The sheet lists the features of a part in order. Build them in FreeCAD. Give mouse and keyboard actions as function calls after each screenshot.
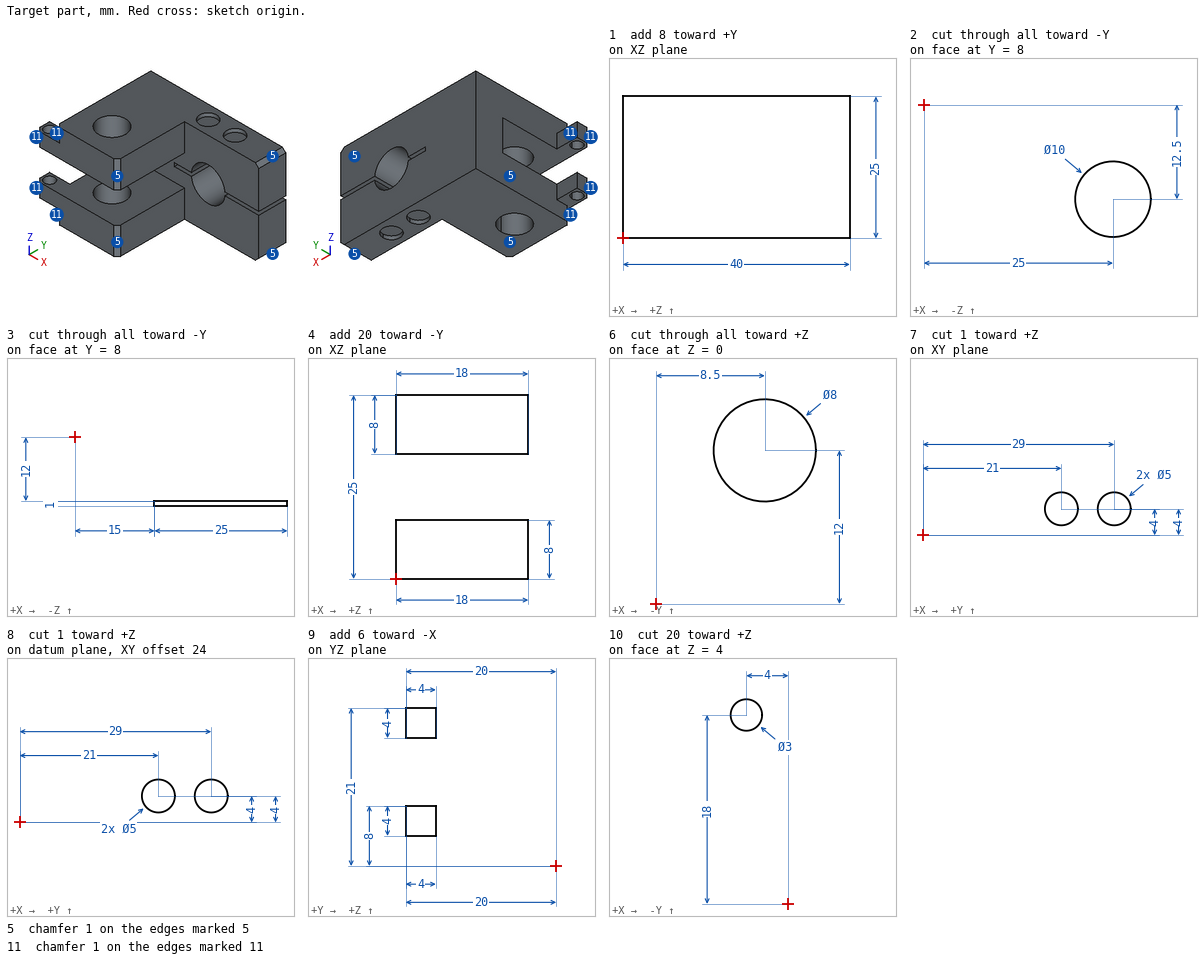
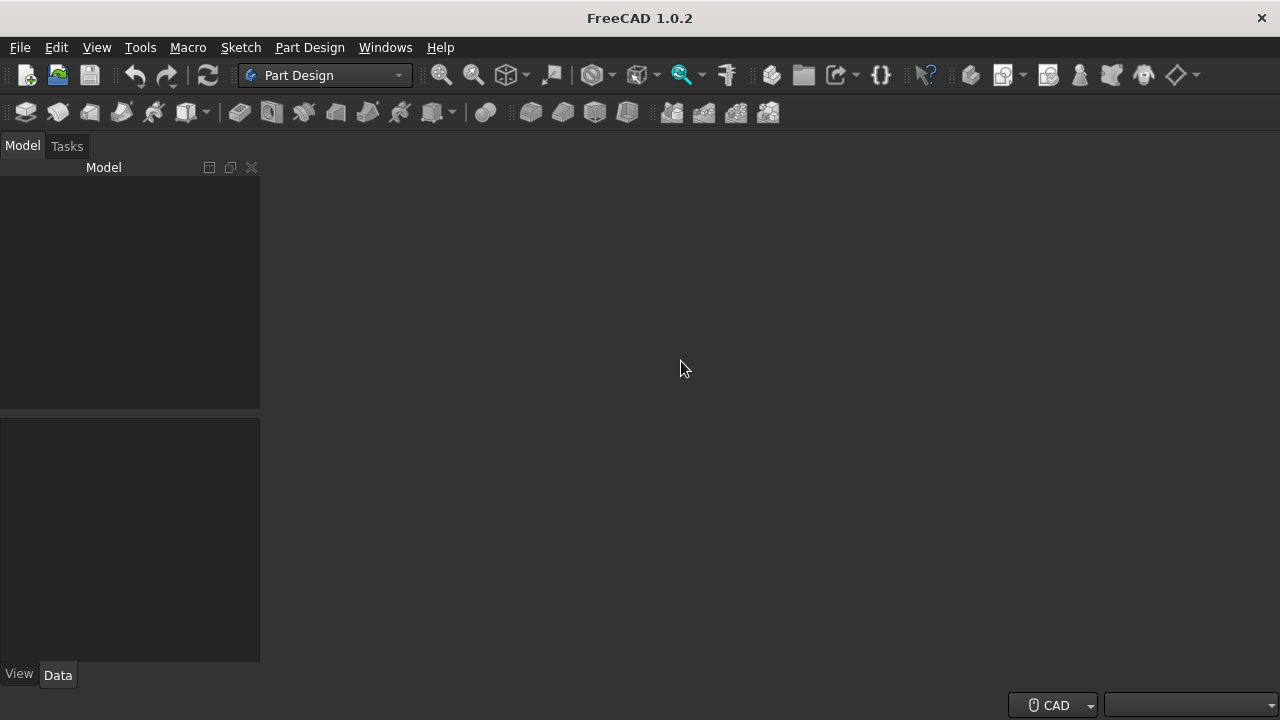
click(26, 76)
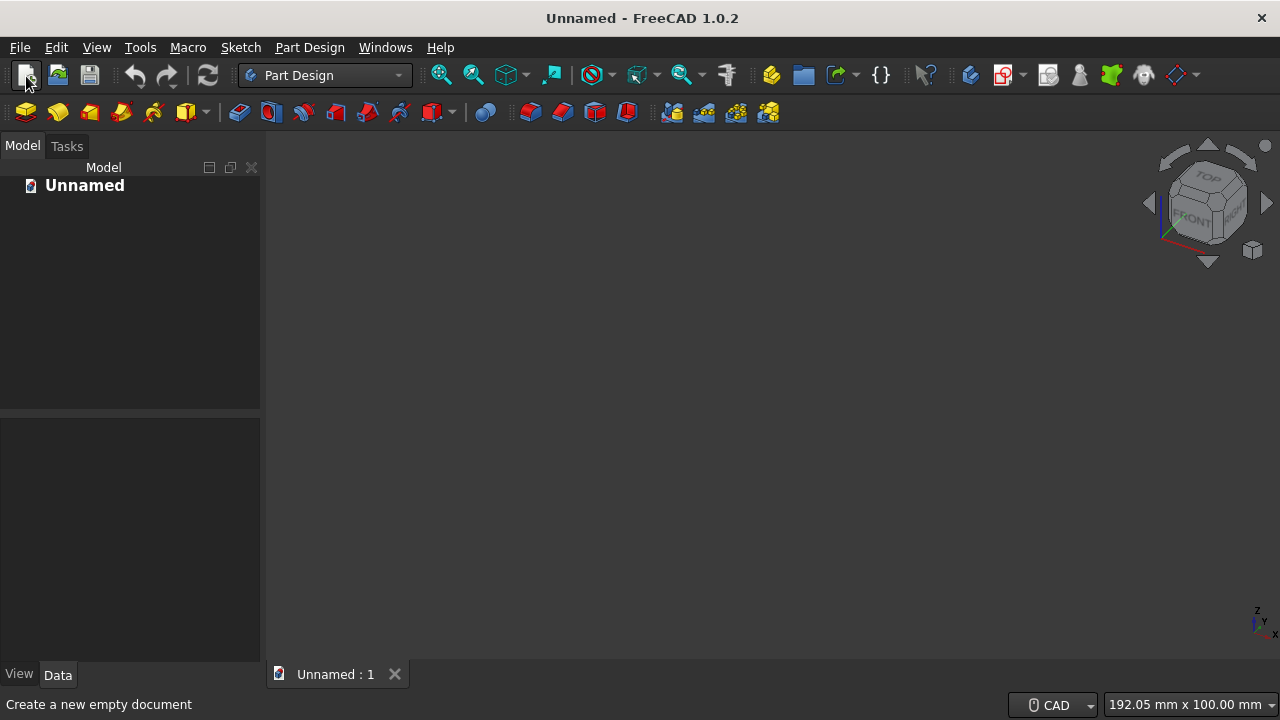
click(1004, 76)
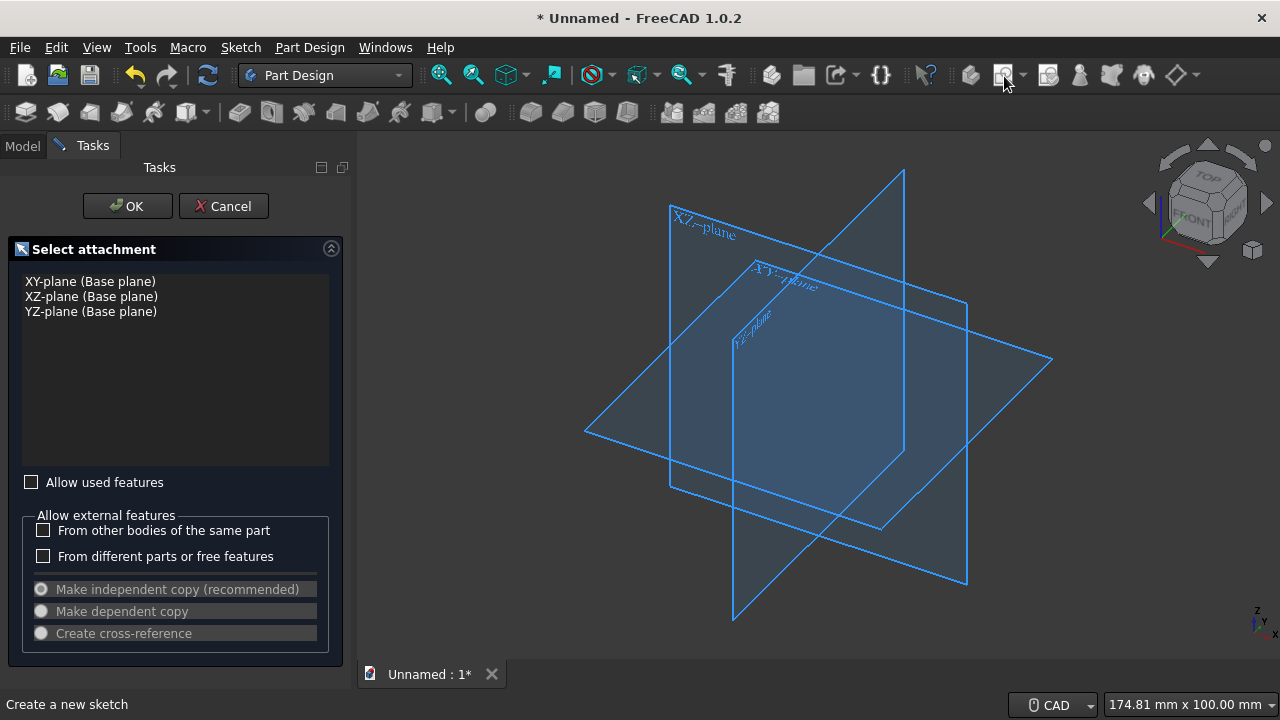
click(82, 296)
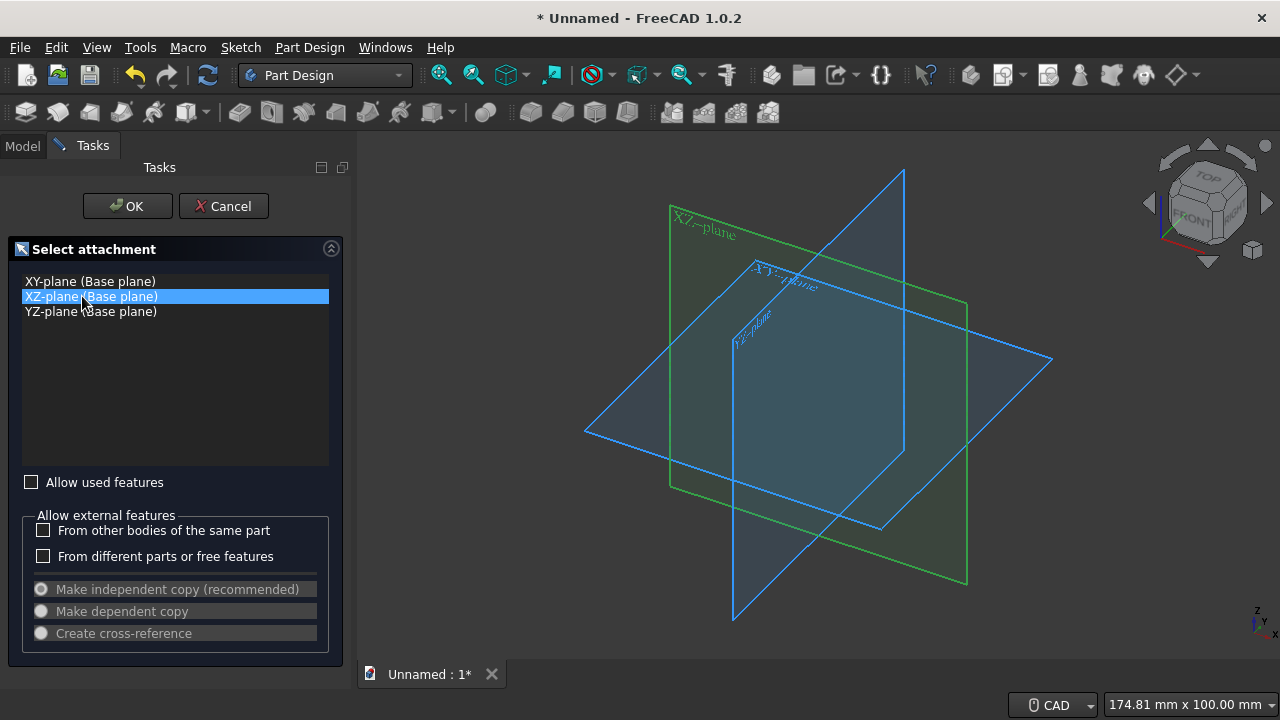
click(128, 206)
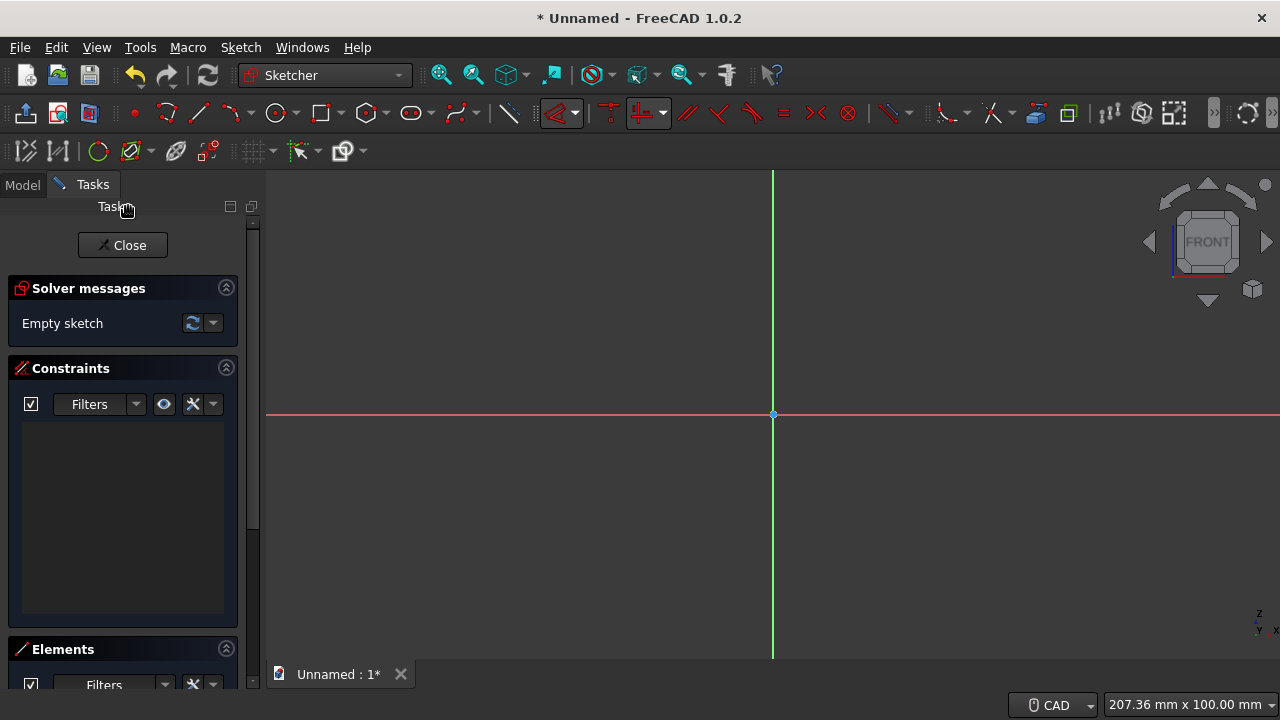
scroll(968, 318, up, 5)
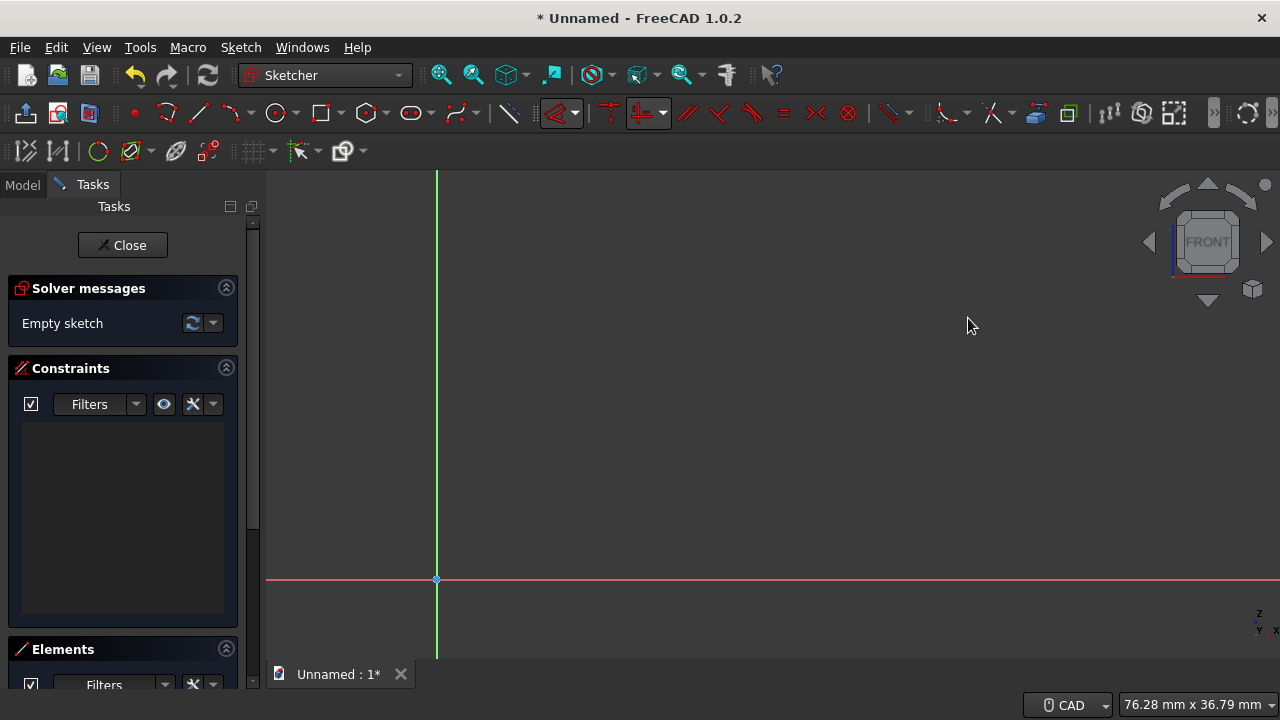
click(322, 114)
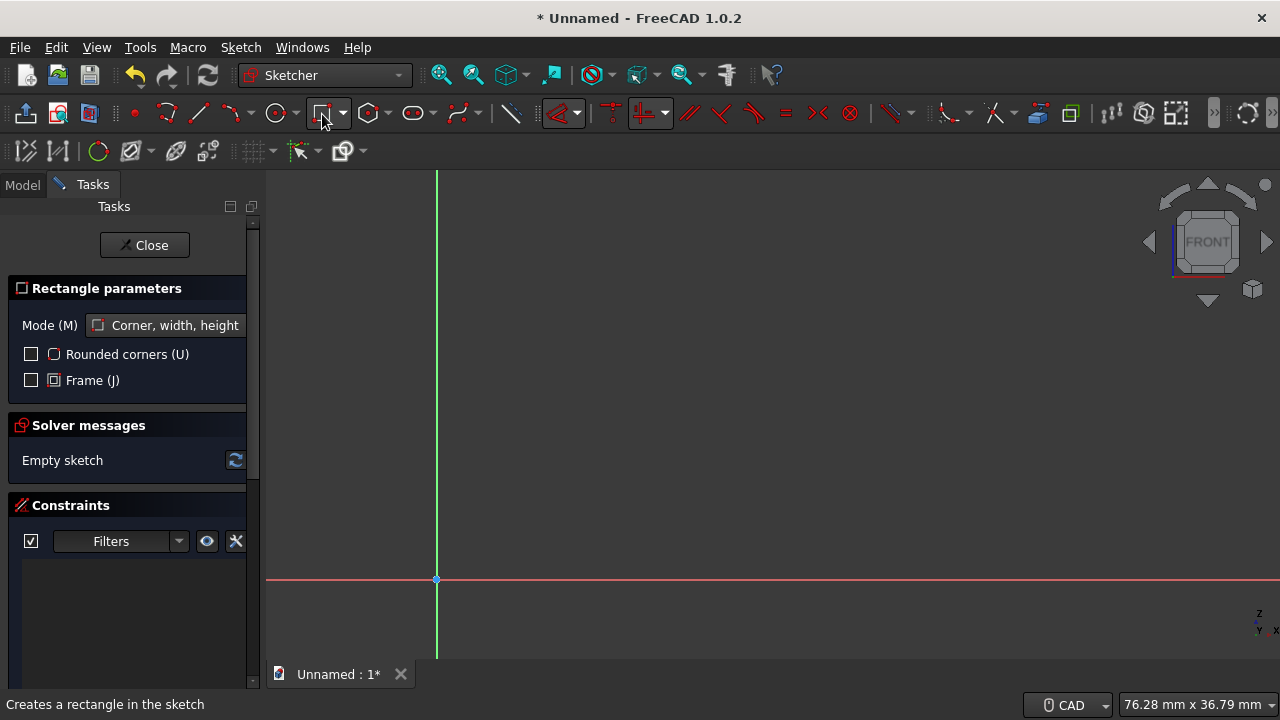
click(437, 580)
click(968, 247)
key(Escape)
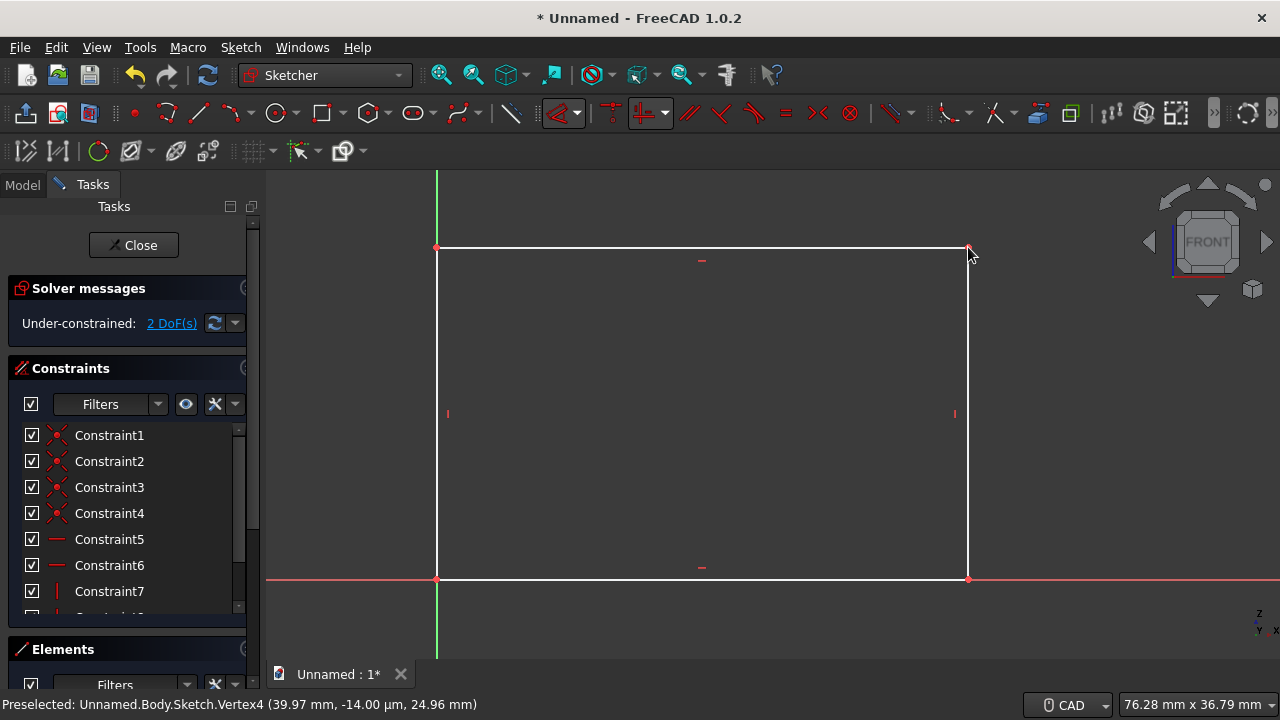
click(558, 114)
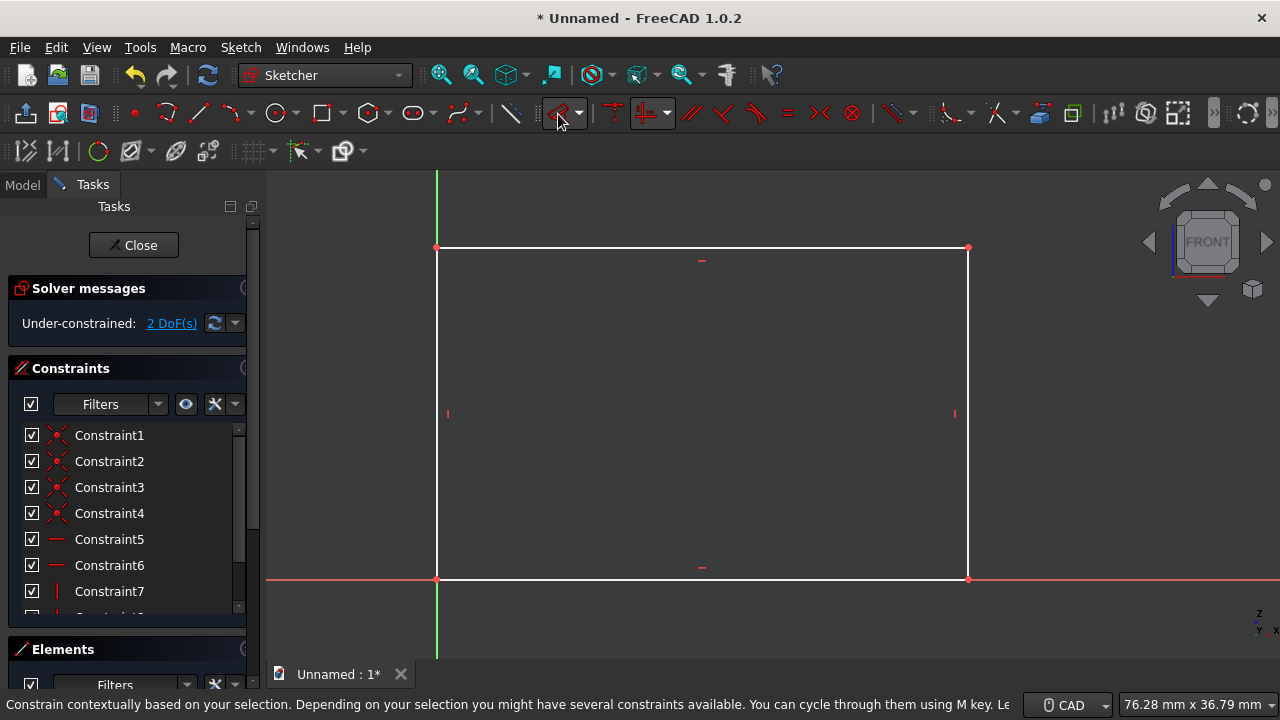
click(596, 580)
click(702, 614)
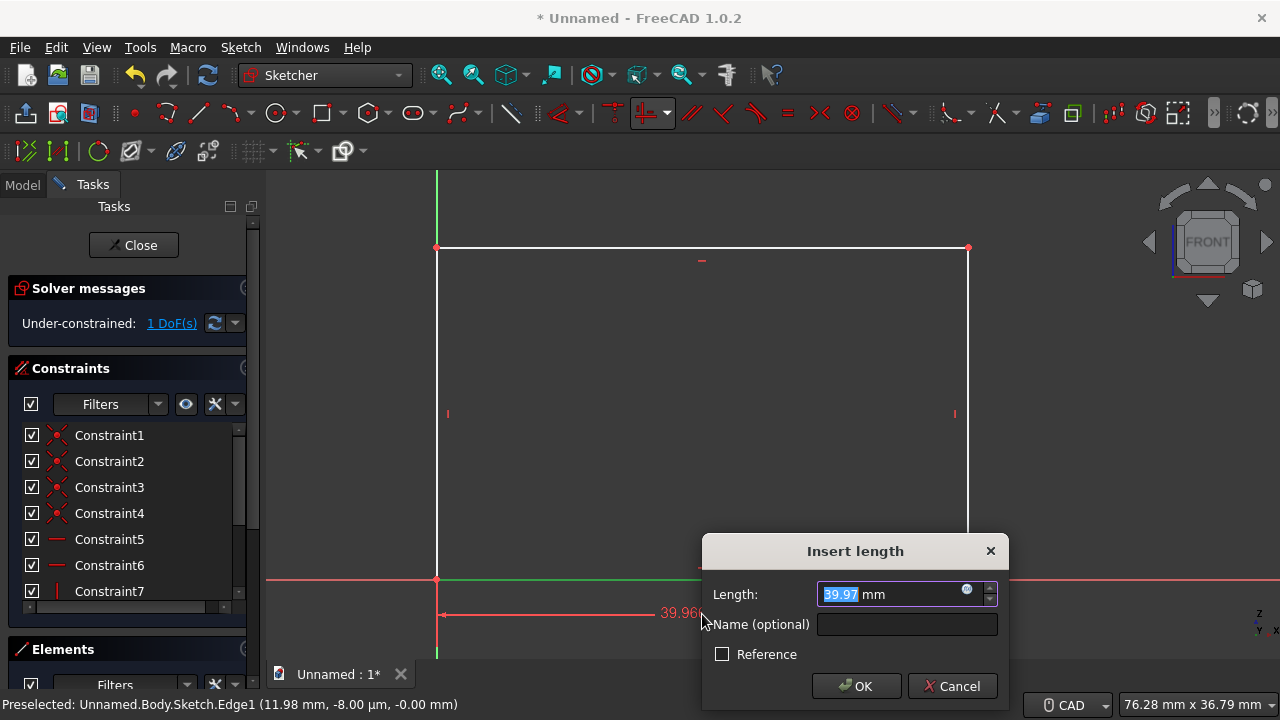
text(40)
key(Return)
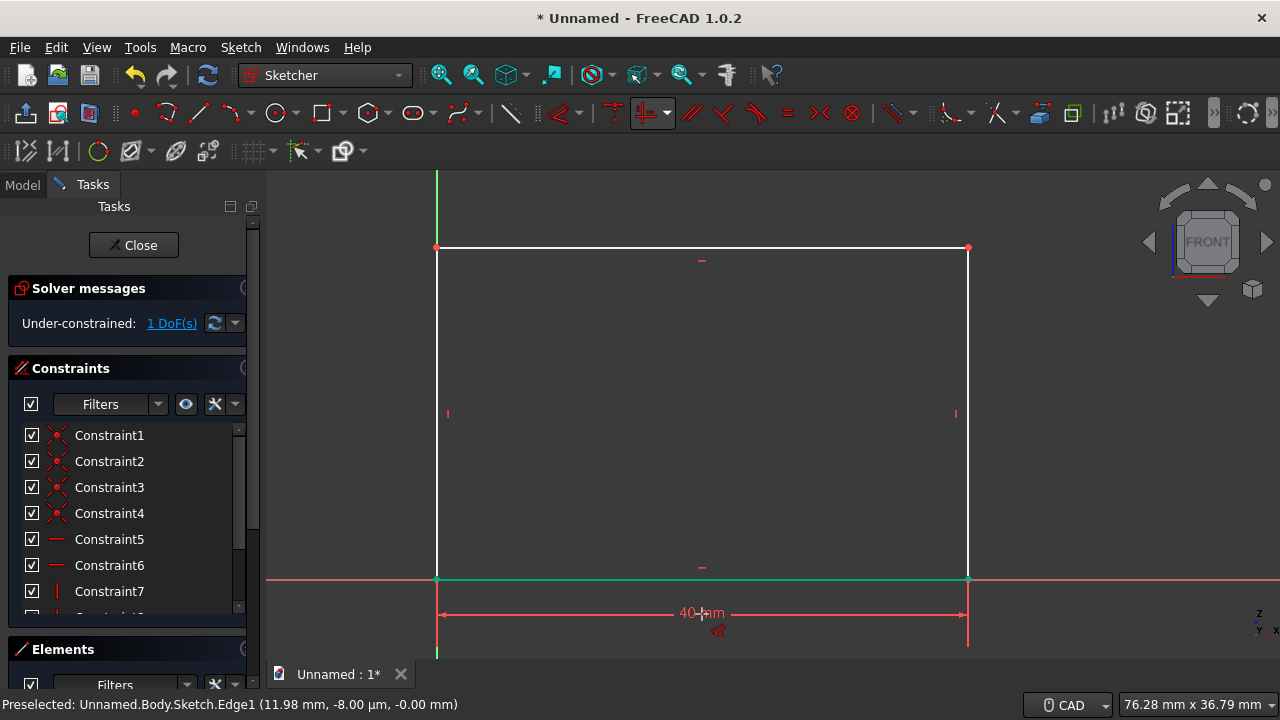
click(968, 480)
click(1002, 414)